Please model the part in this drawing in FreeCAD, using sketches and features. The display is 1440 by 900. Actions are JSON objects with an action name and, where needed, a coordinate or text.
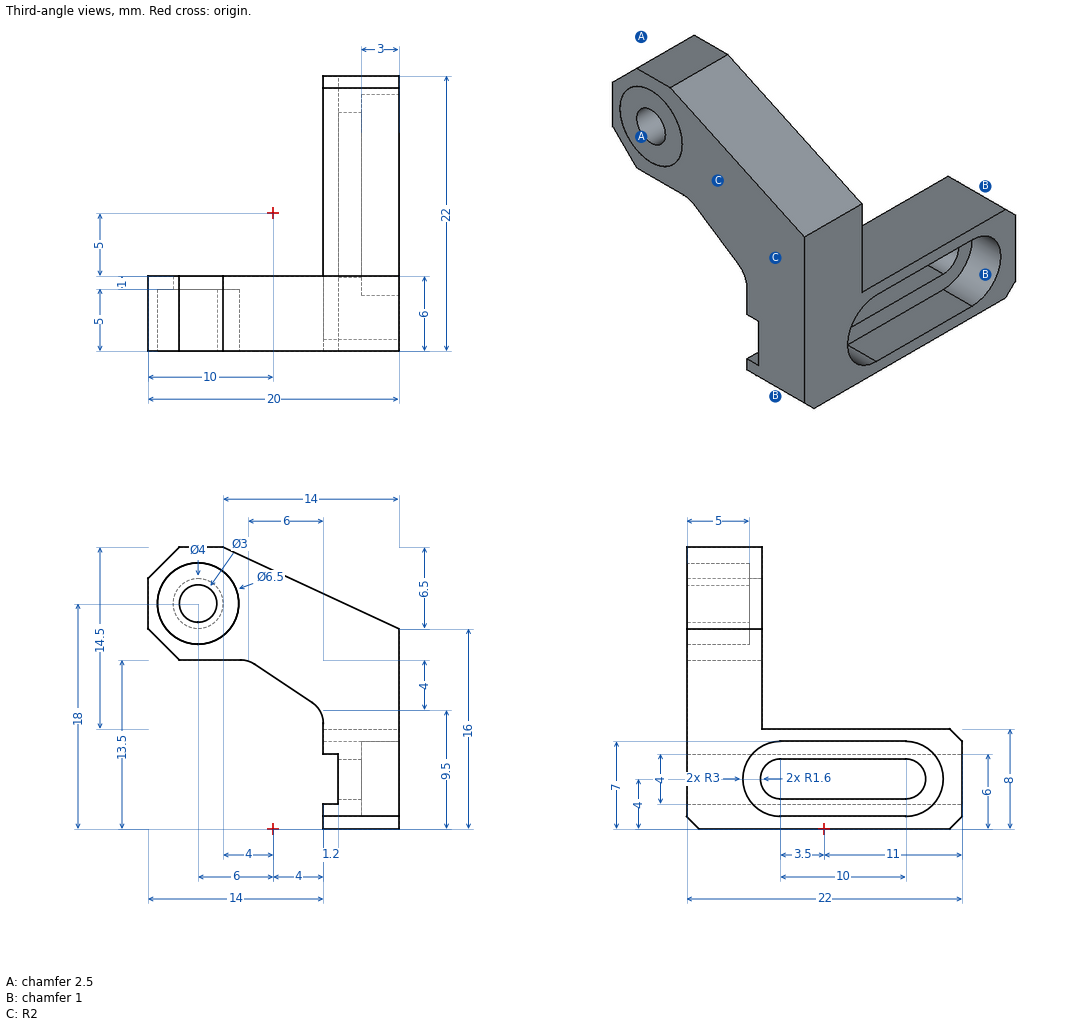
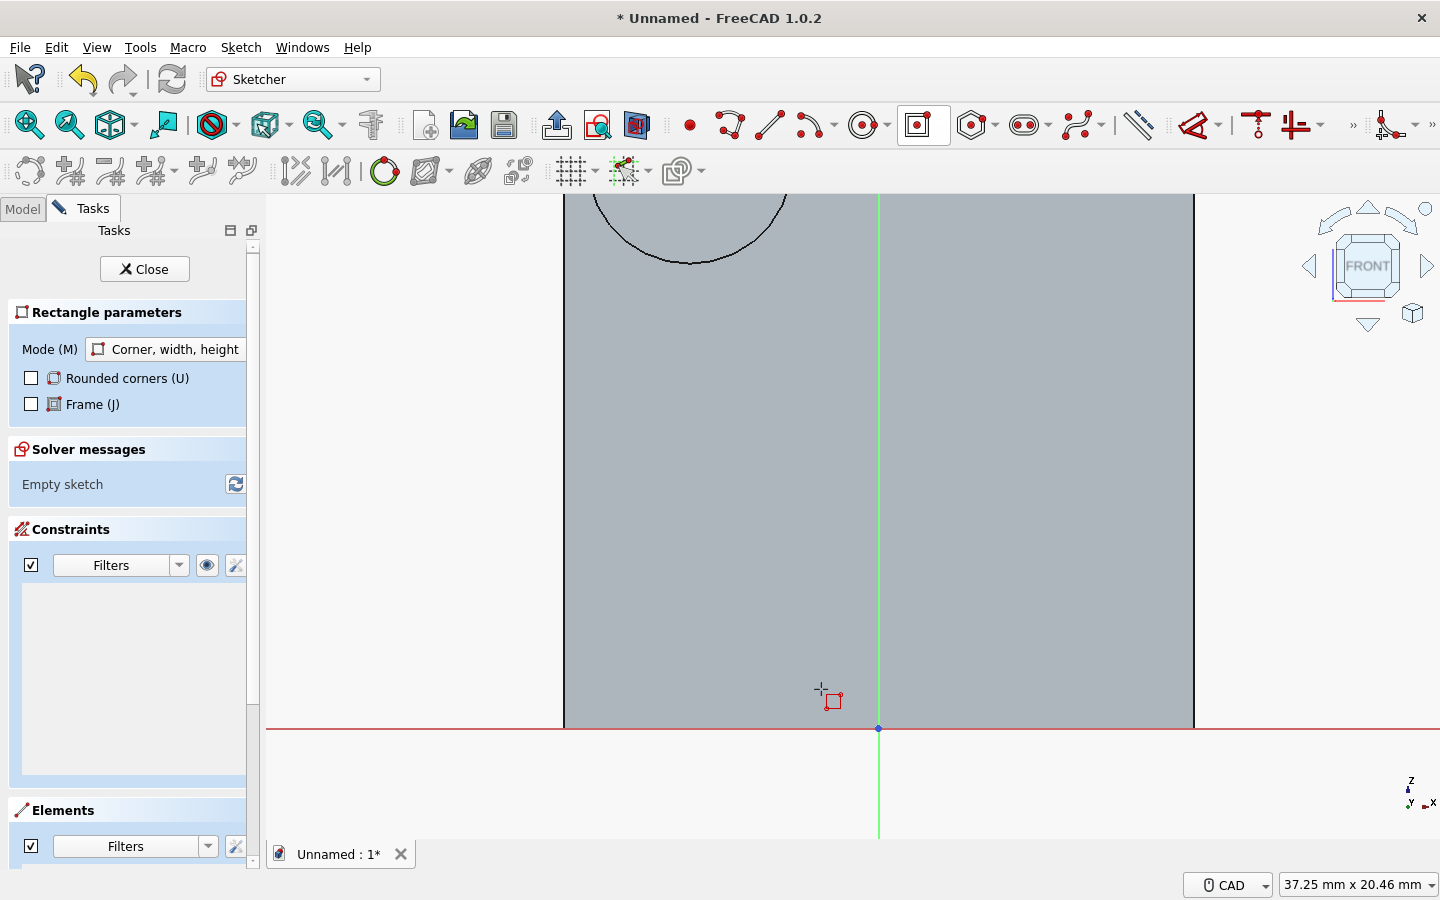
{"action": "left_click", "coordinate": [564, 303]}
{"action": "left_click", "coordinate": [1005, 729]}
{"action": "key", "text": "Escape"}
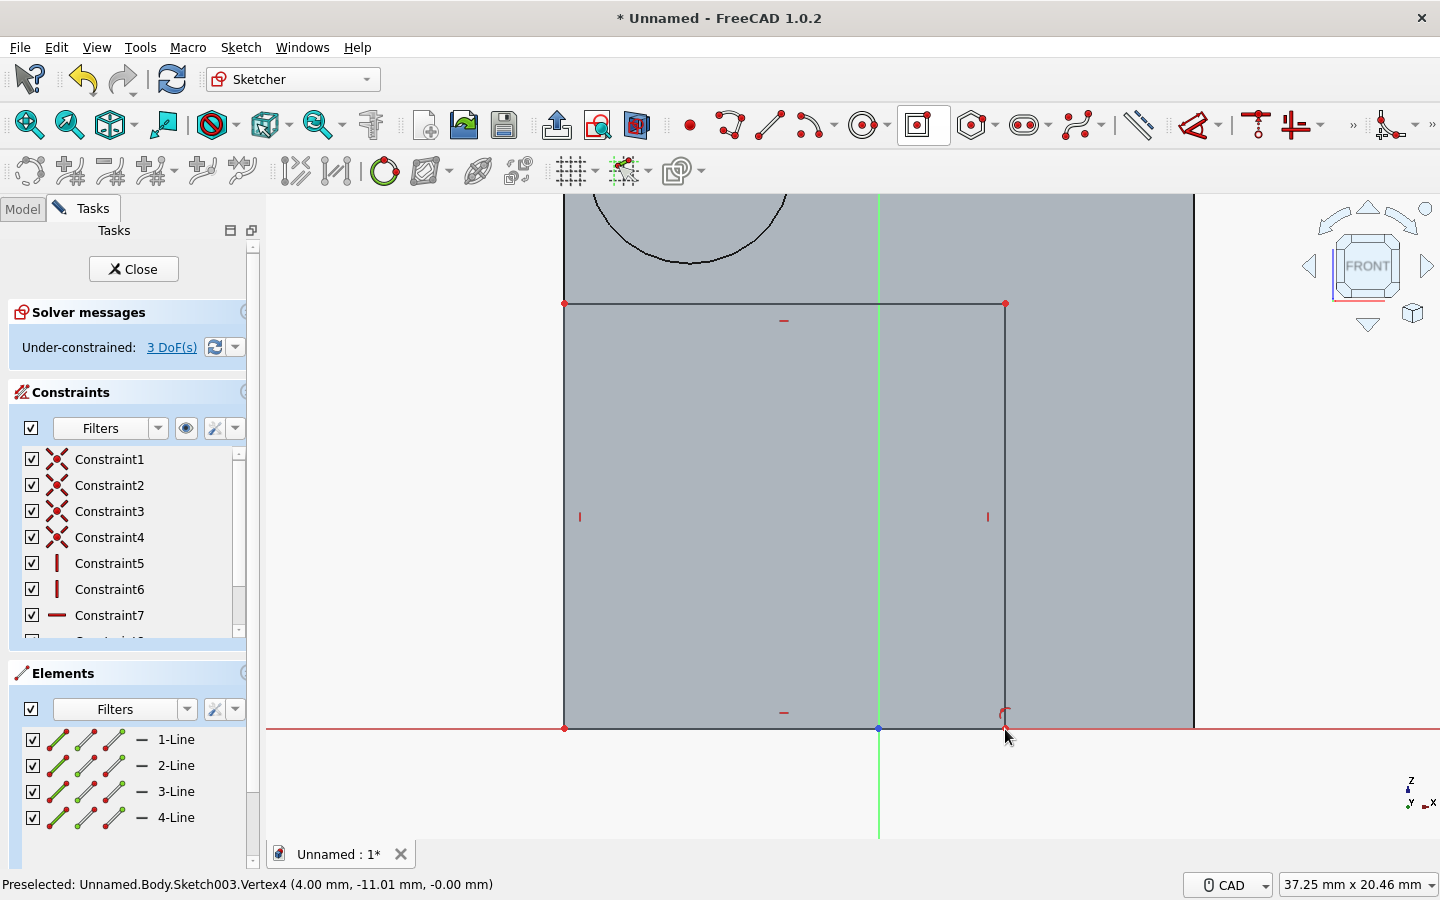
{"action": "left_click", "coordinate": [1194, 126]}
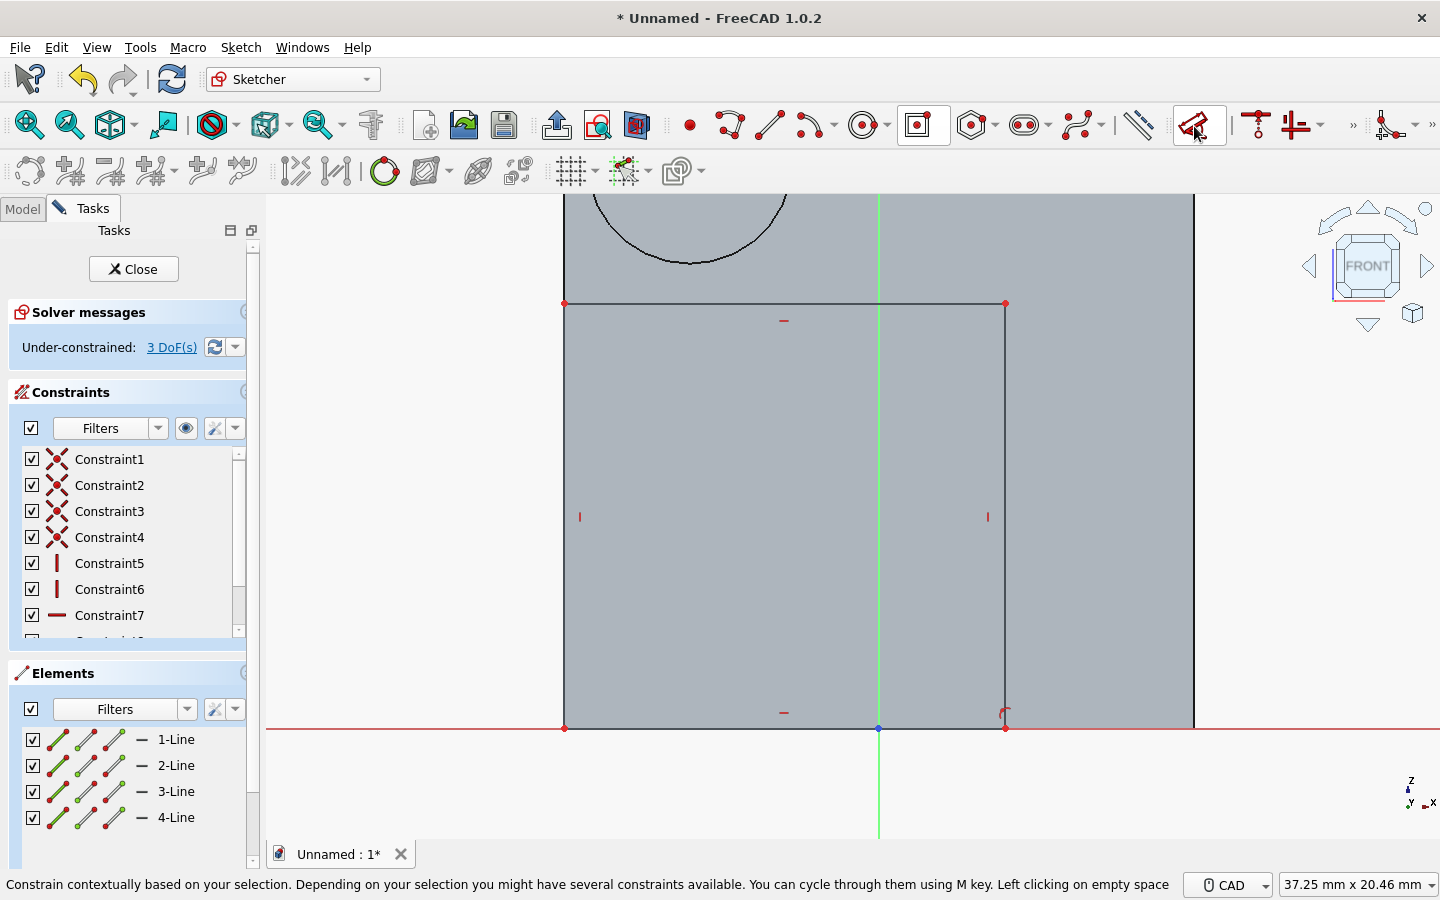
{"action": "left_click", "coordinate": [696, 729]}
{"action": "left_click", "coordinate": [785, 763]}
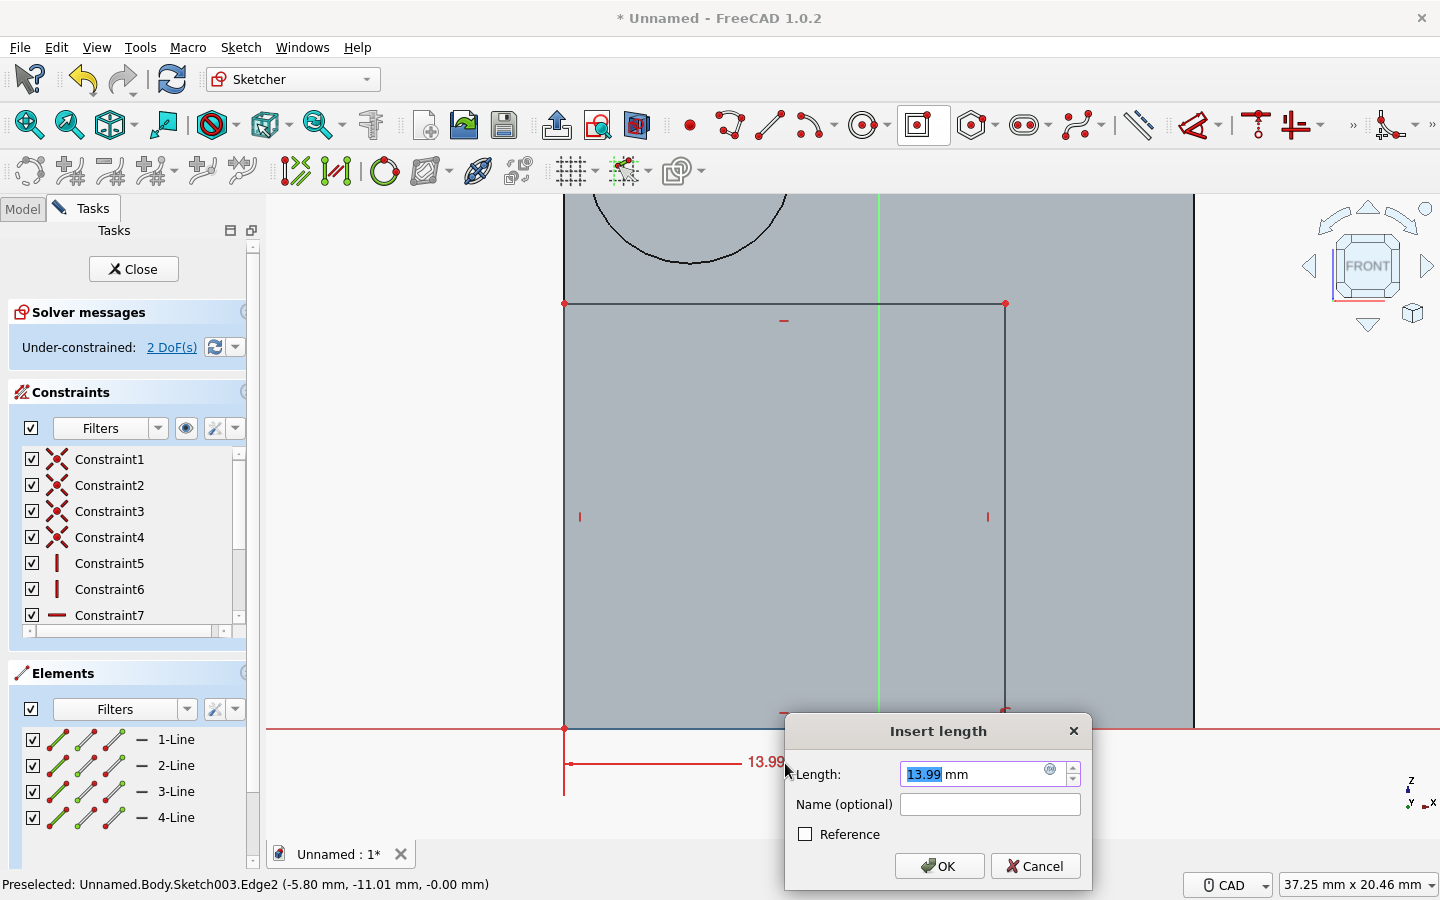
{"action": "type", "text": "14"}
{"action": "key", "text": "Return"}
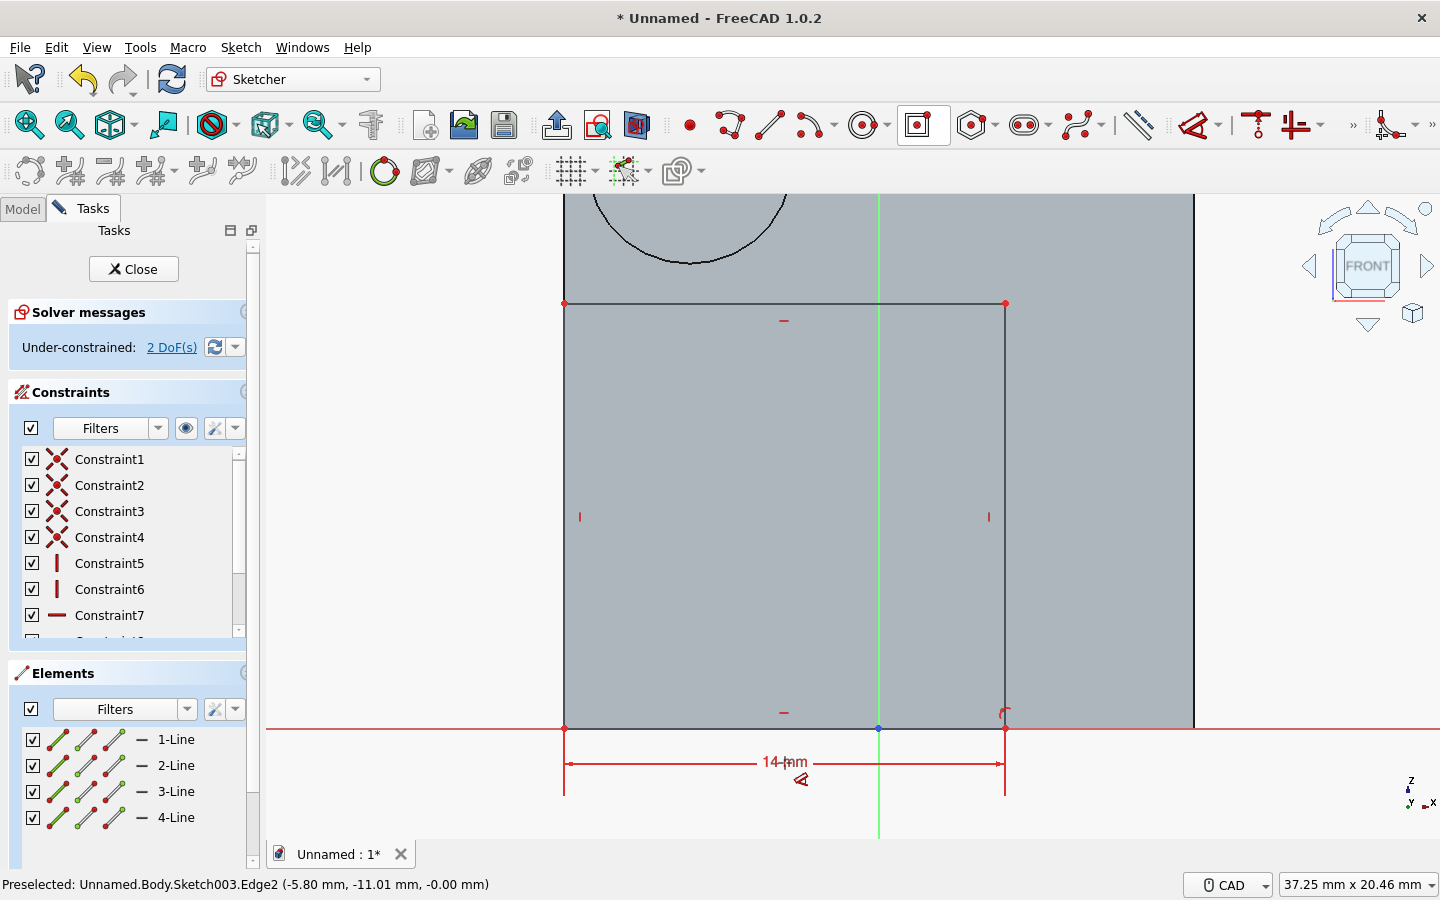
{"action": "left_click", "coordinate": [1005, 729]}
{"action": "left_click", "coordinate": [942, 763]}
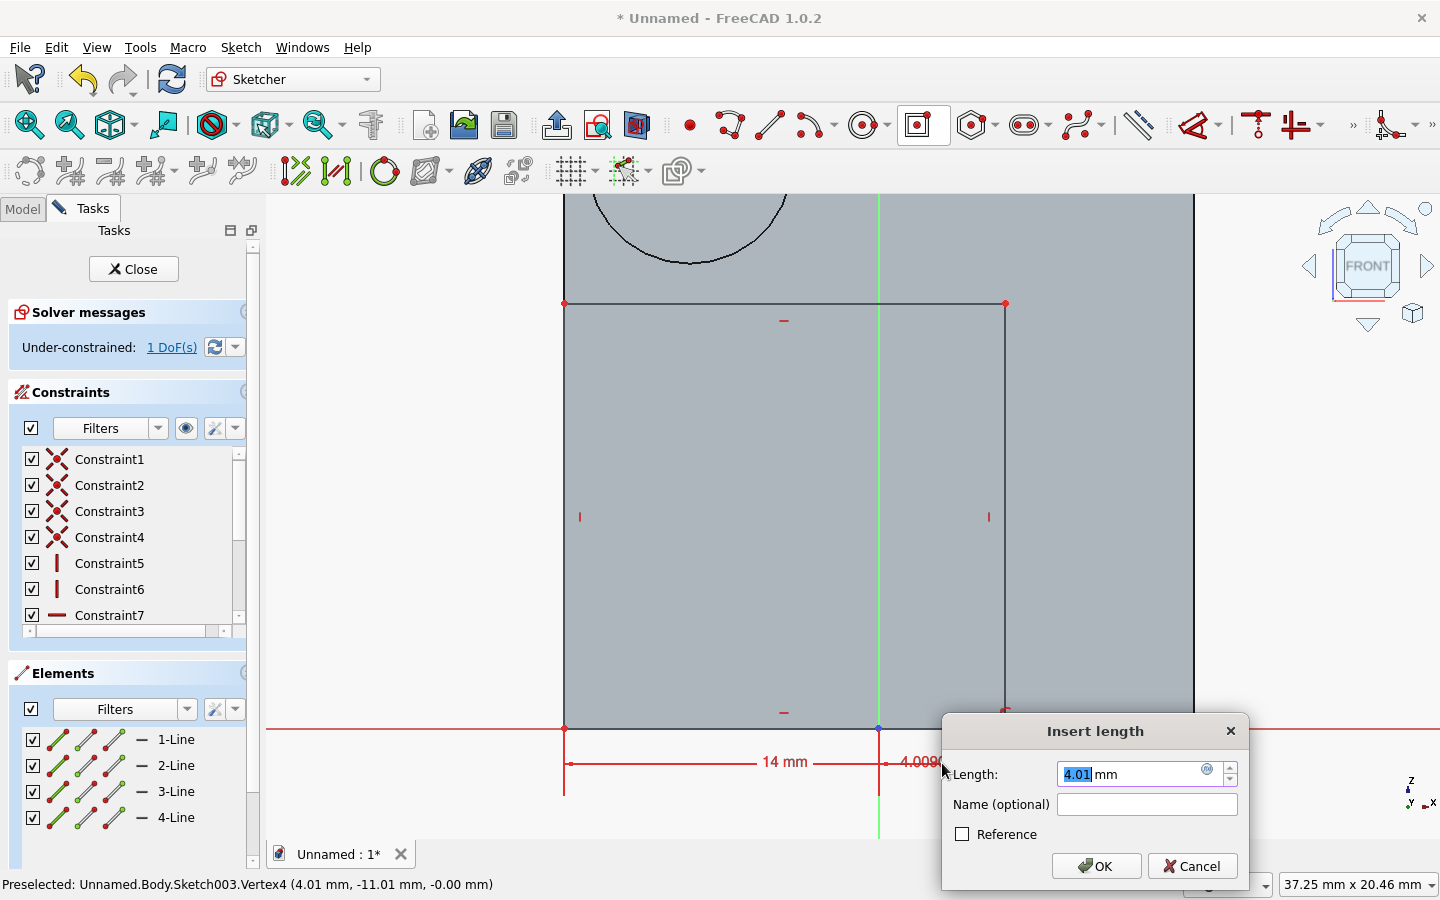
{"action": "type", "text": "4"}
{"action": "key", "text": "Return"}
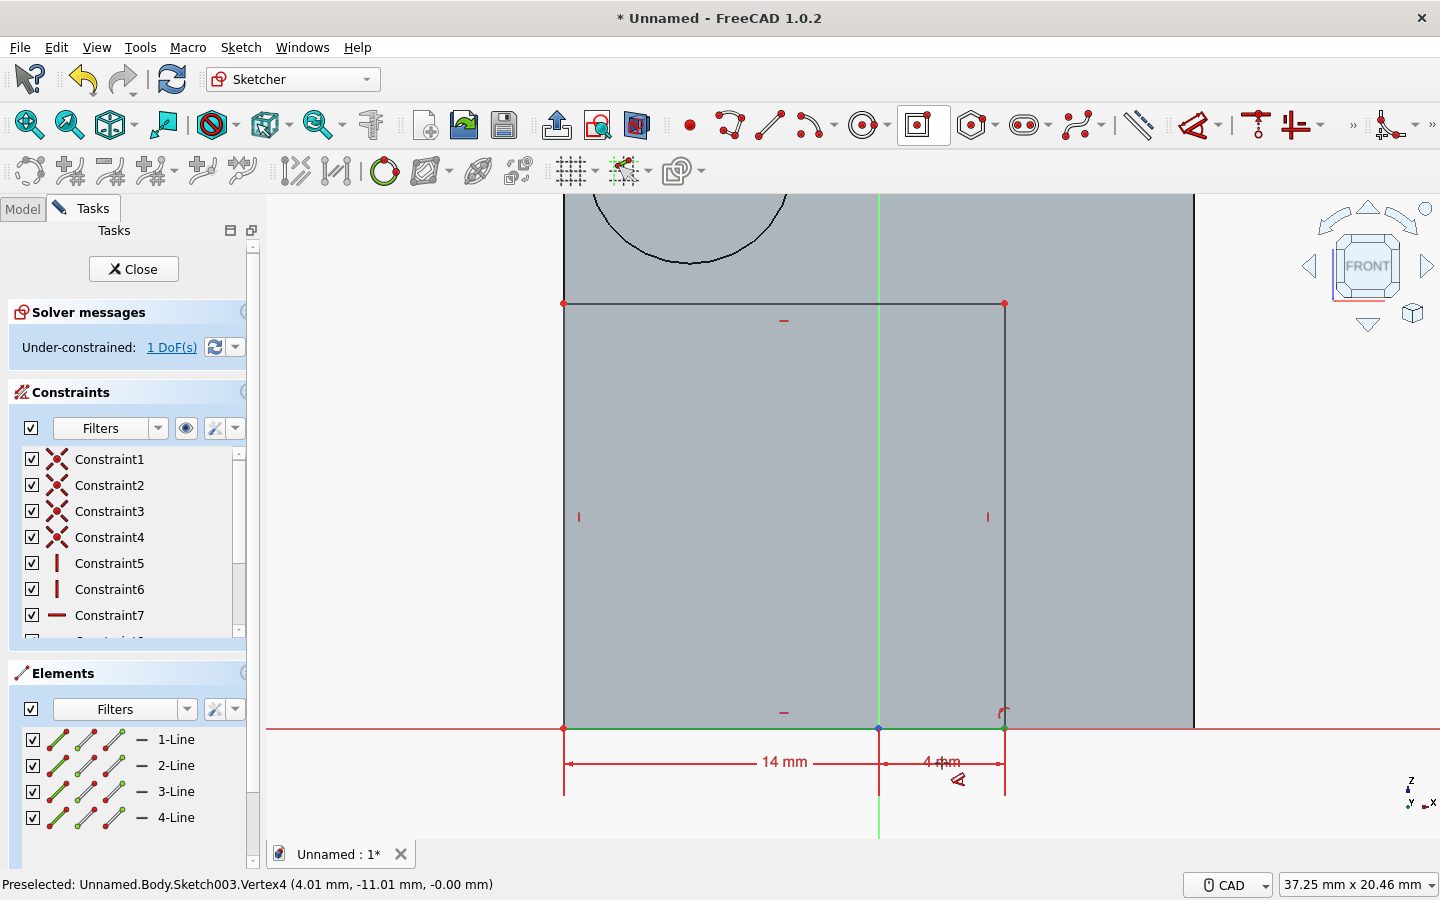
{"action": "left_click", "coordinate": [564, 431]}
{"action": "left_click", "coordinate": [530, 516]}